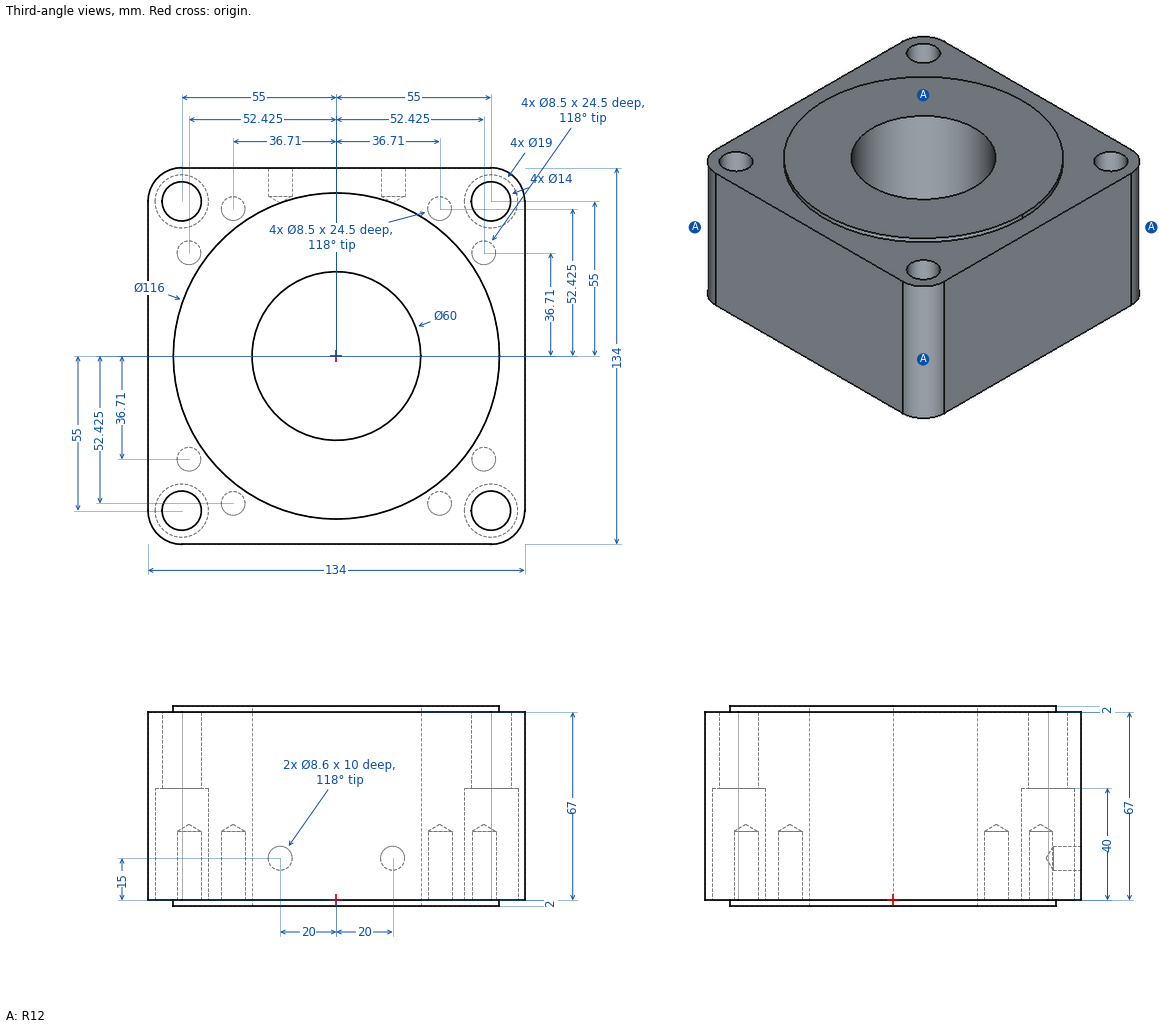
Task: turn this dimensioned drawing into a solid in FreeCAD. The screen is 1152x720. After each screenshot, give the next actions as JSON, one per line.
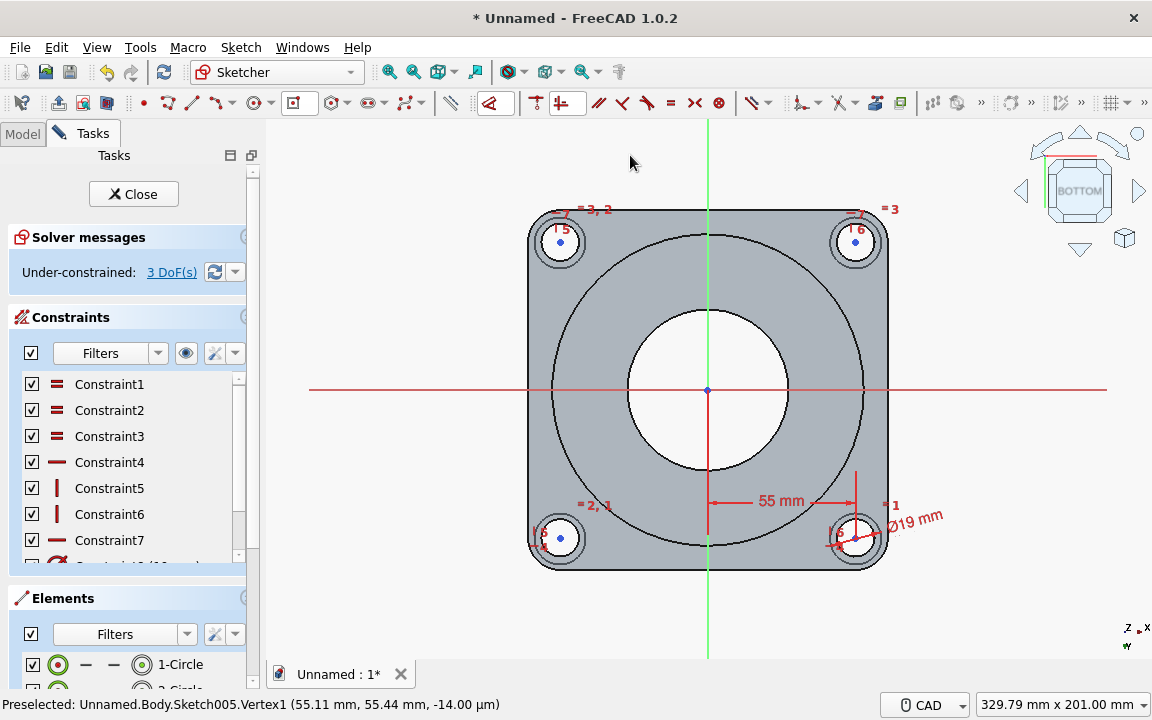
{"action": "left_click", "coordinate": [856, 539]}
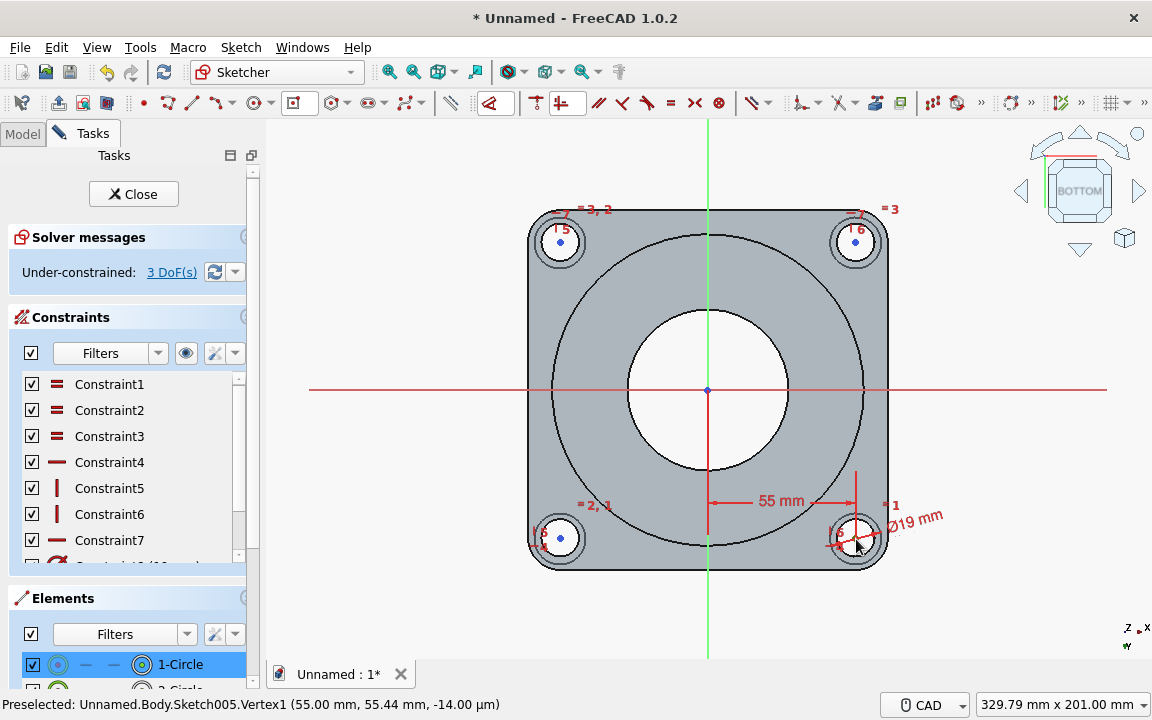
{"action": "left_click", "coordinate": [508, 104]}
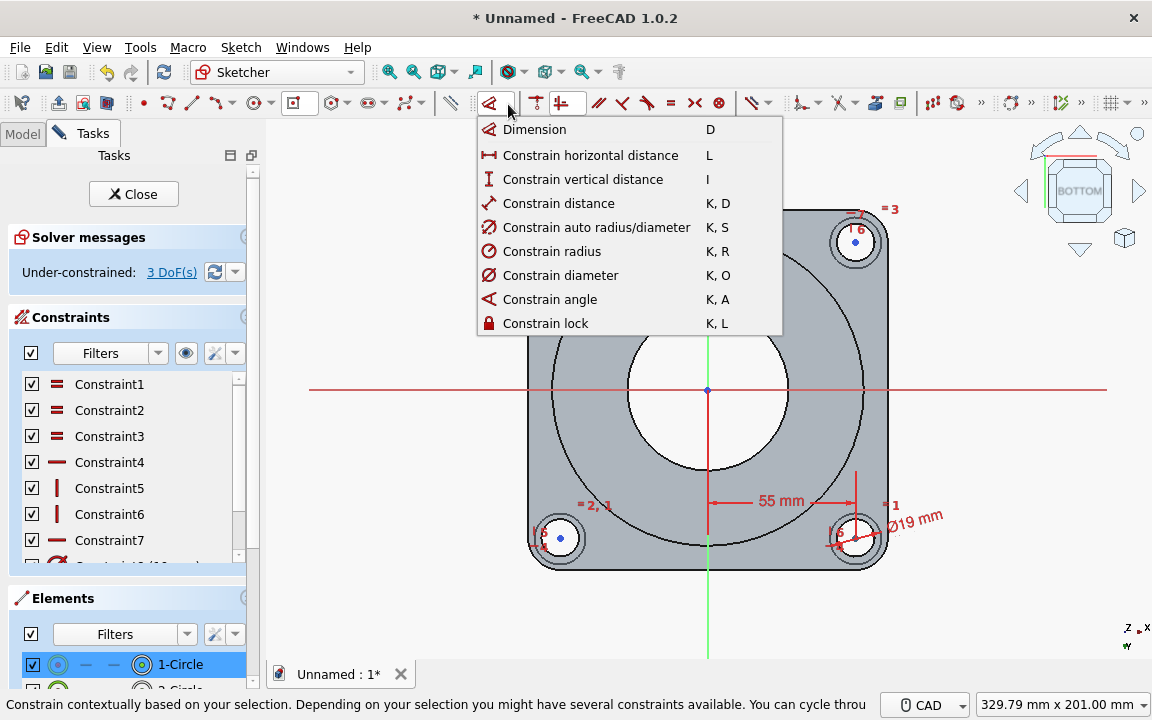
{"action": "left_click", "coordinate": [630, 179]}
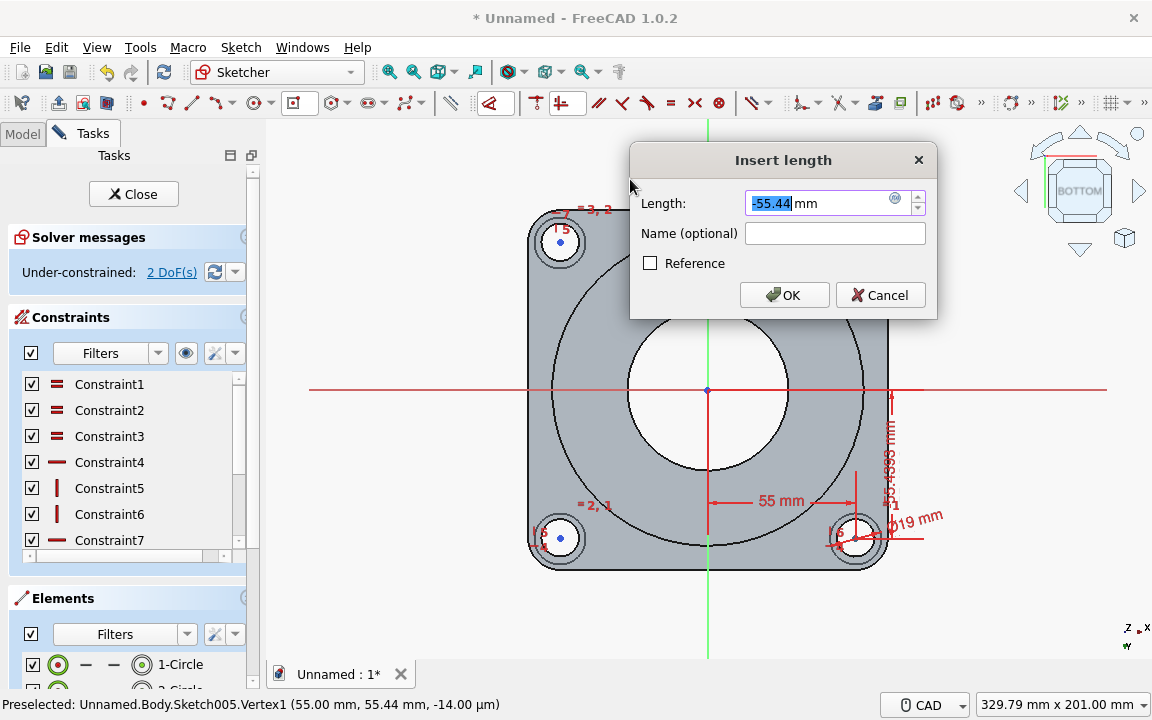
{"action": "type", "text": "-55"}
{"action": "key", "text": "Return"}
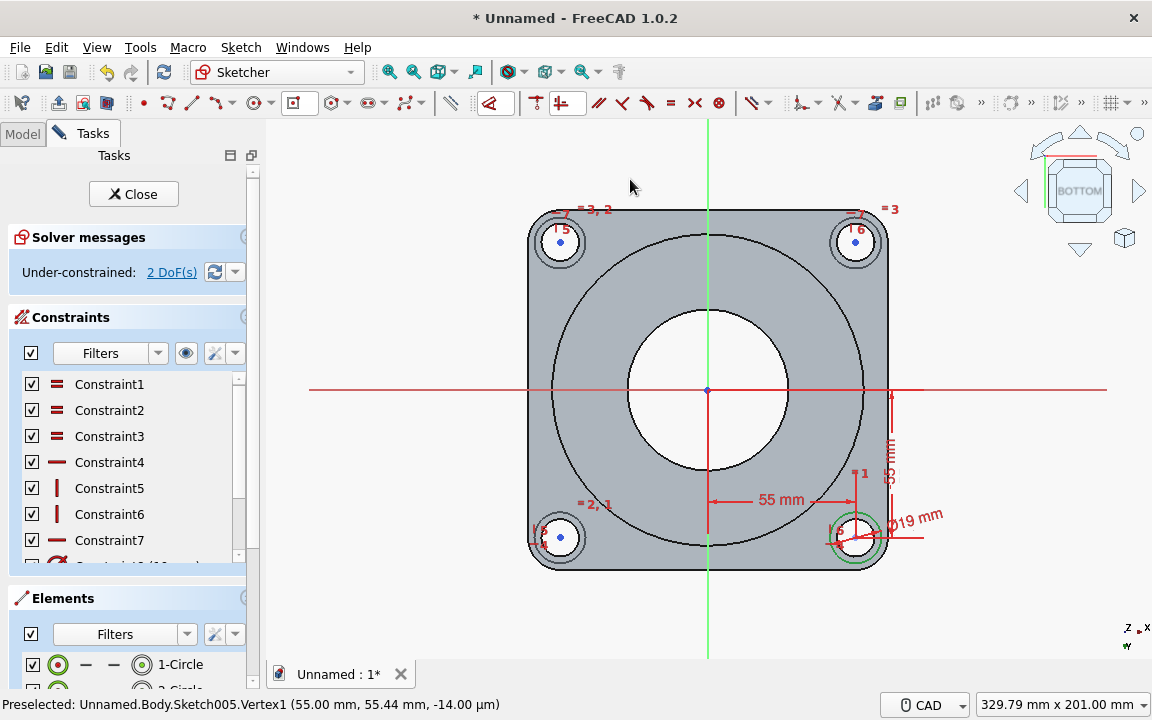
{"action": "left_click", "coordinate": [560, 538]}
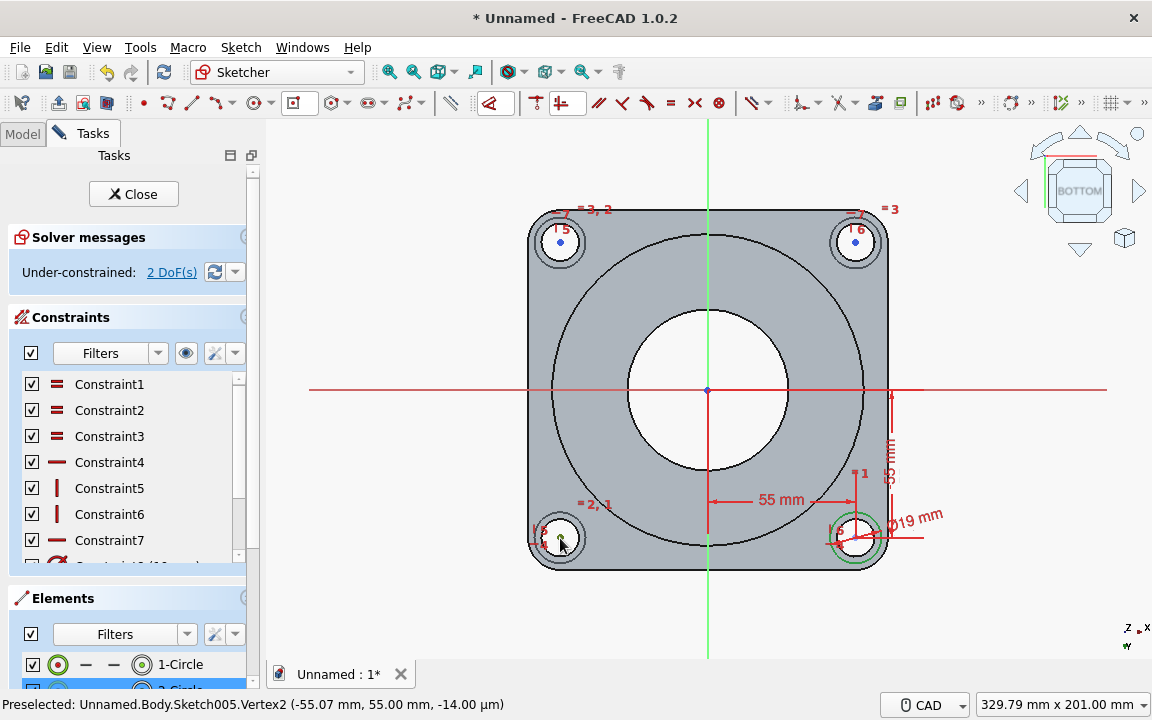
{"action": "left_click", "coordinate": [508, 104]}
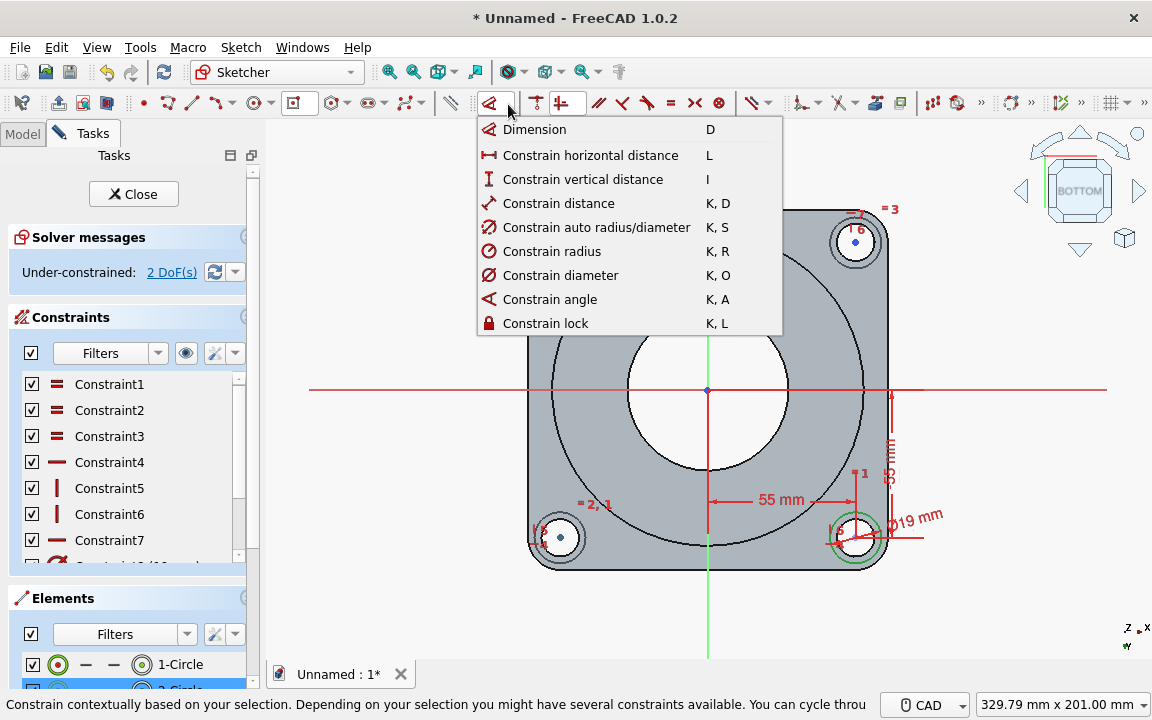
{"action": "left_click", "coordinate": [630, 155]}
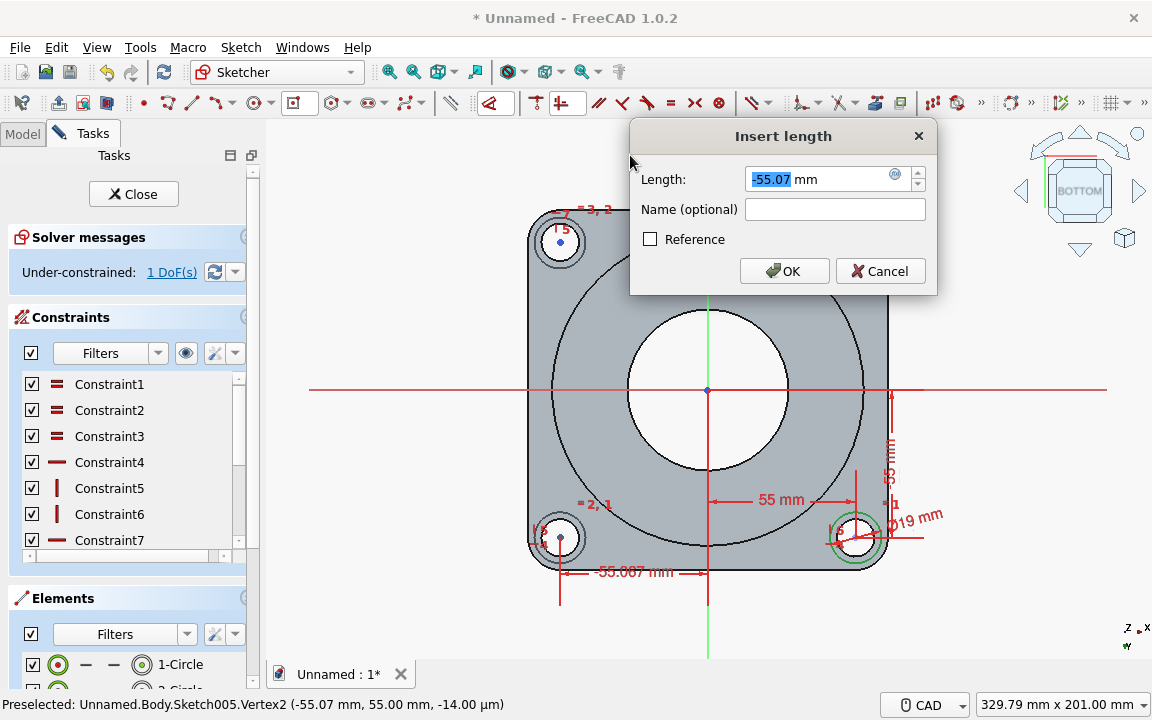
{"action": "type", "text": "-55"}
{"action": "key", "text": "Return"}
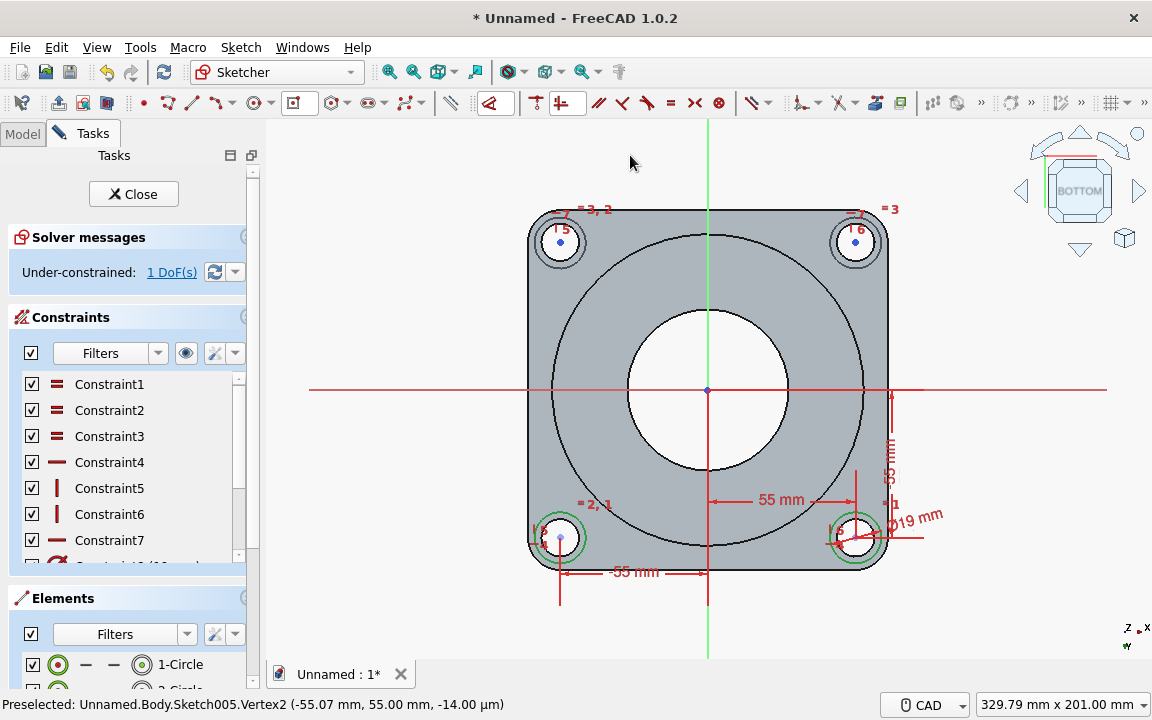
{"action": "left_click", "coordinate": [560, 243]}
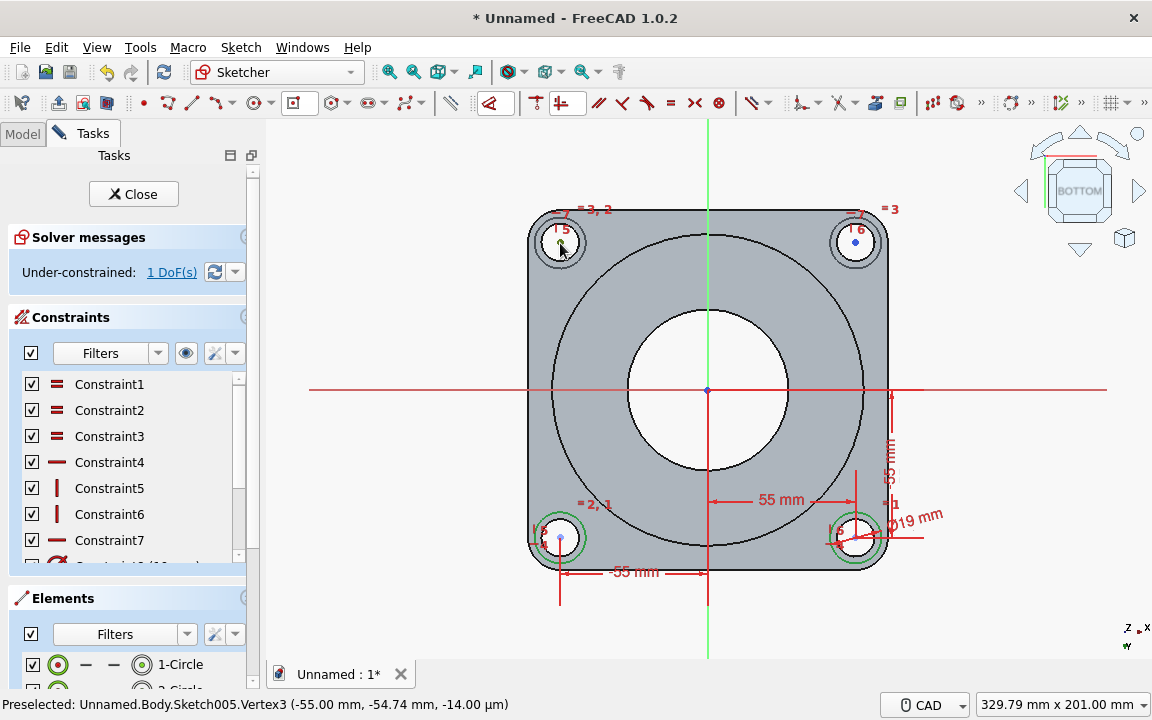
{"action": "key", "text": "i"}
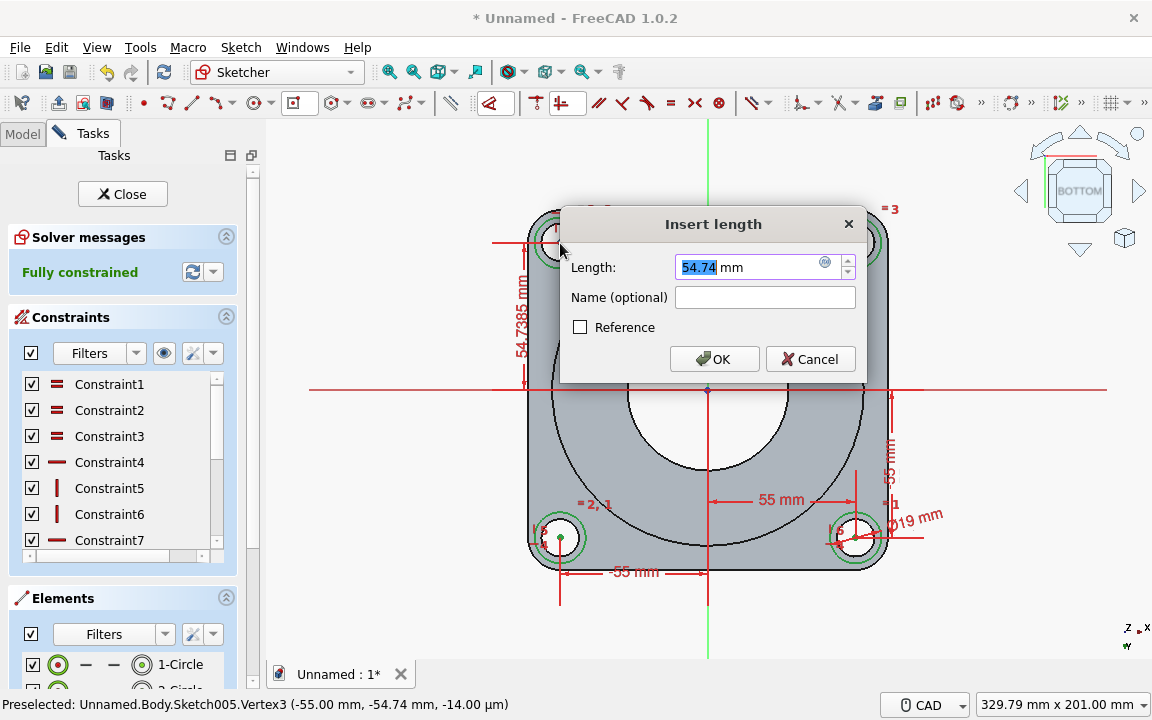
{"action": "type", "text": "55"}
{"action": "key", "text": "Return"}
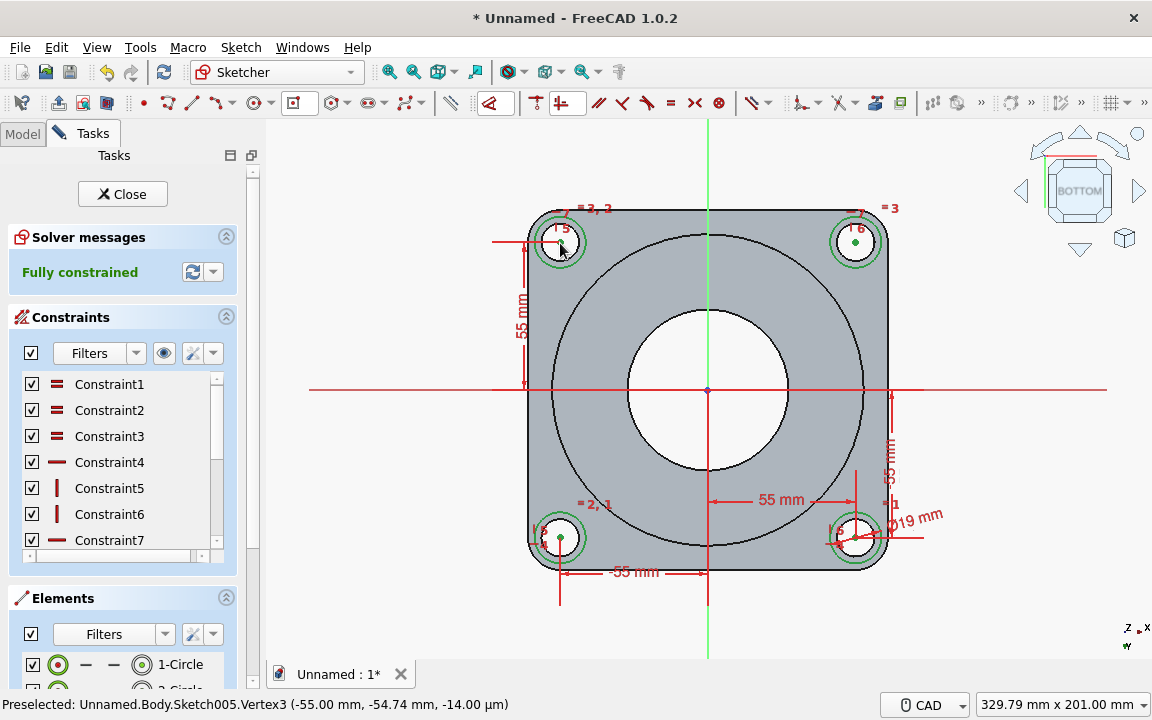
{"action": "left_click", "coordinate": [123, 194]}